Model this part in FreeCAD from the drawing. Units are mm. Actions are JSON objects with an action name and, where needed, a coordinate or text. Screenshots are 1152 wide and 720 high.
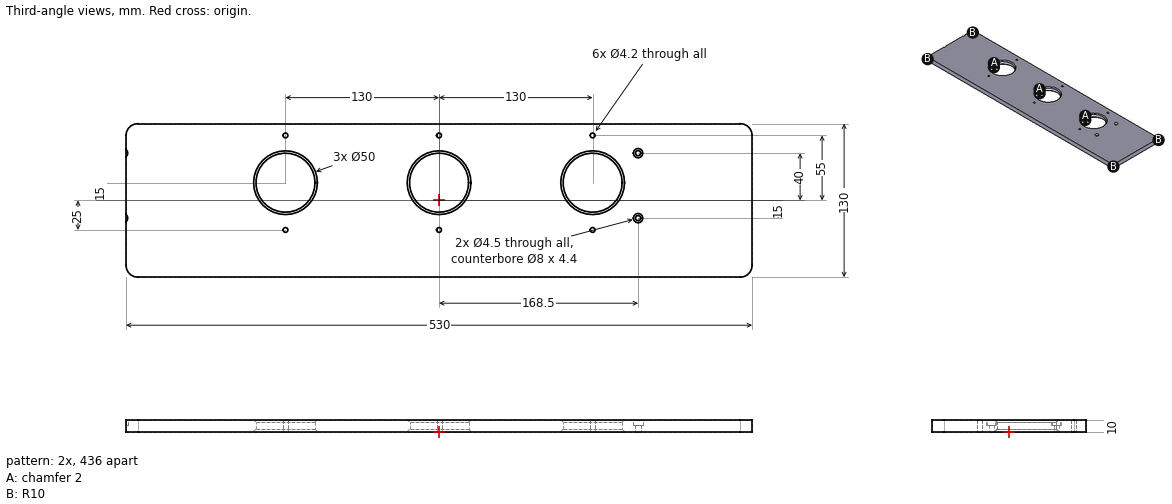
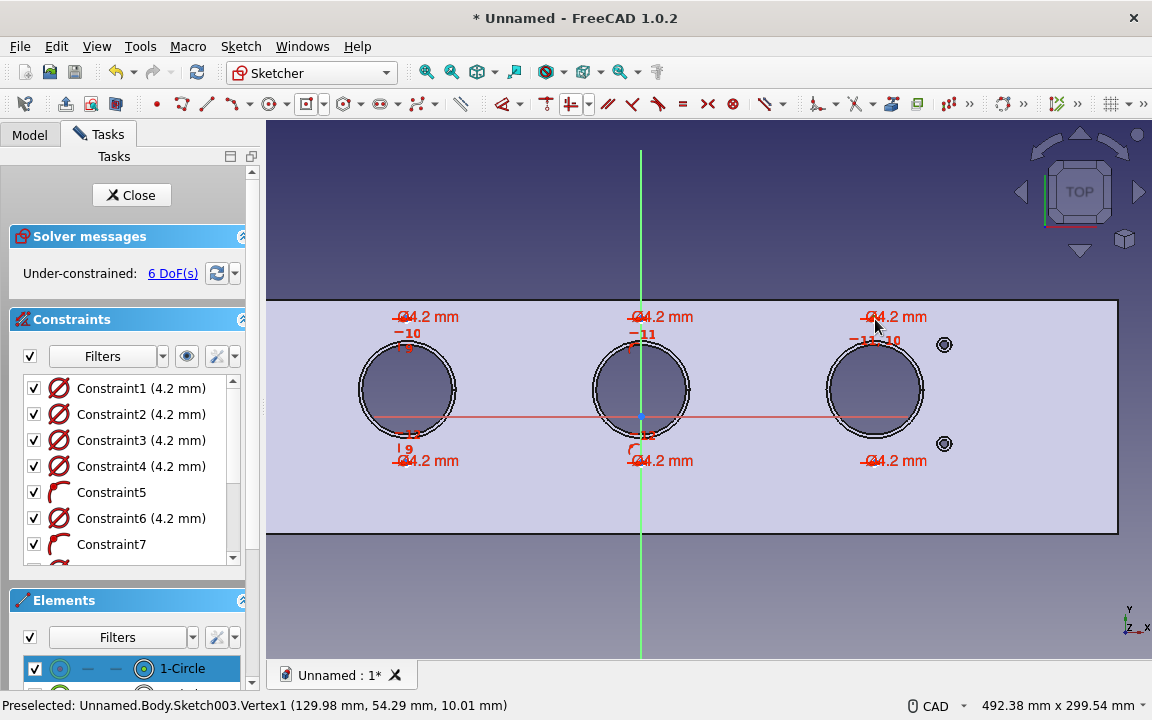
{"action": "left_click", "coordinate": [875, 463]}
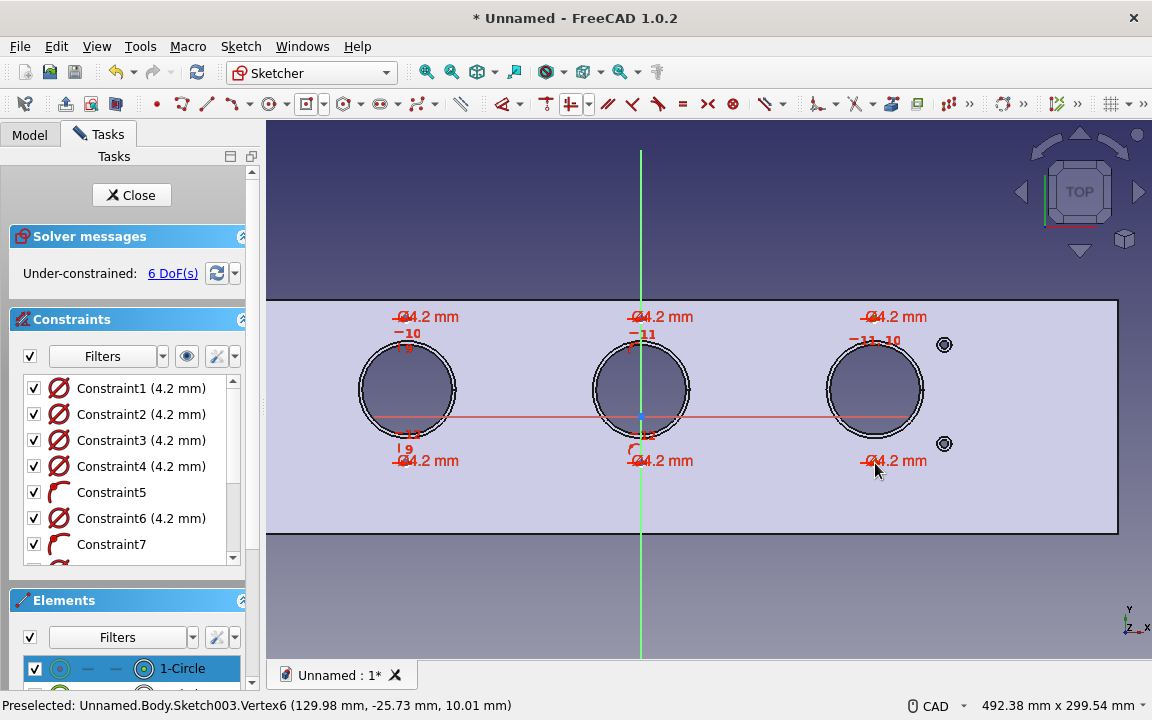
{"action": "left_click", "coordinate": [588, 104]}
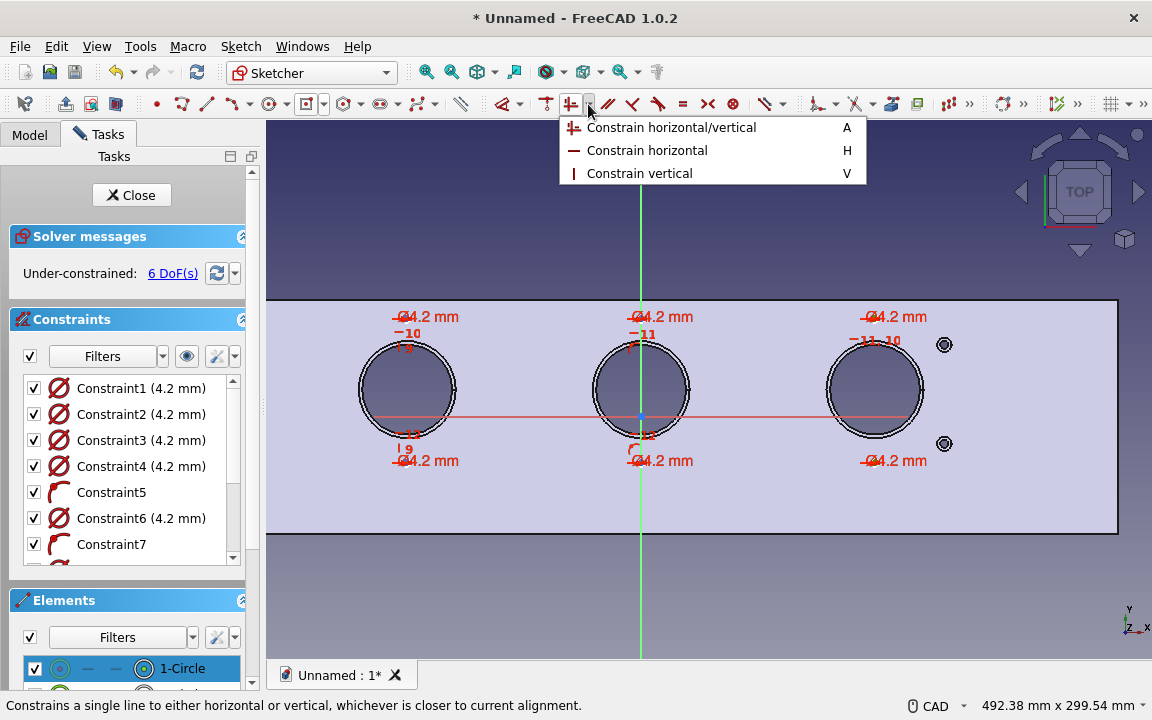
{"action": "left_click", "coordinate": [713, 174]}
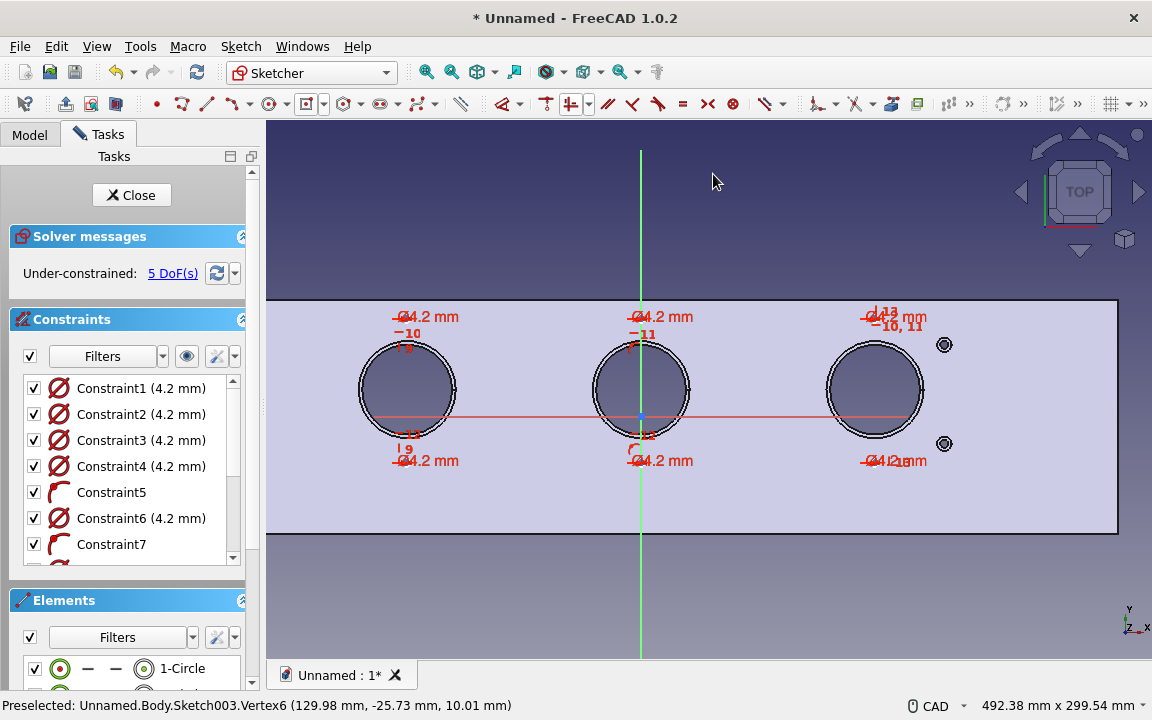
{"action": "left_click", "coordinate": [641, 463]}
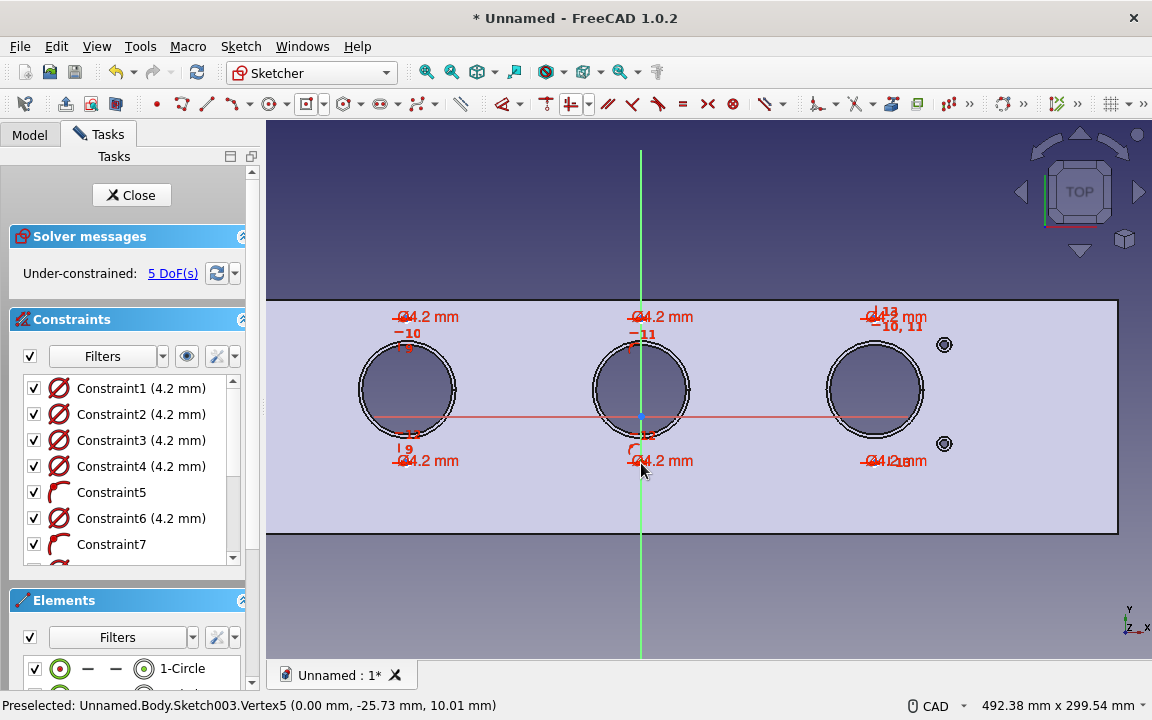
{"action": "left_click", "coordinate": [875, 463]}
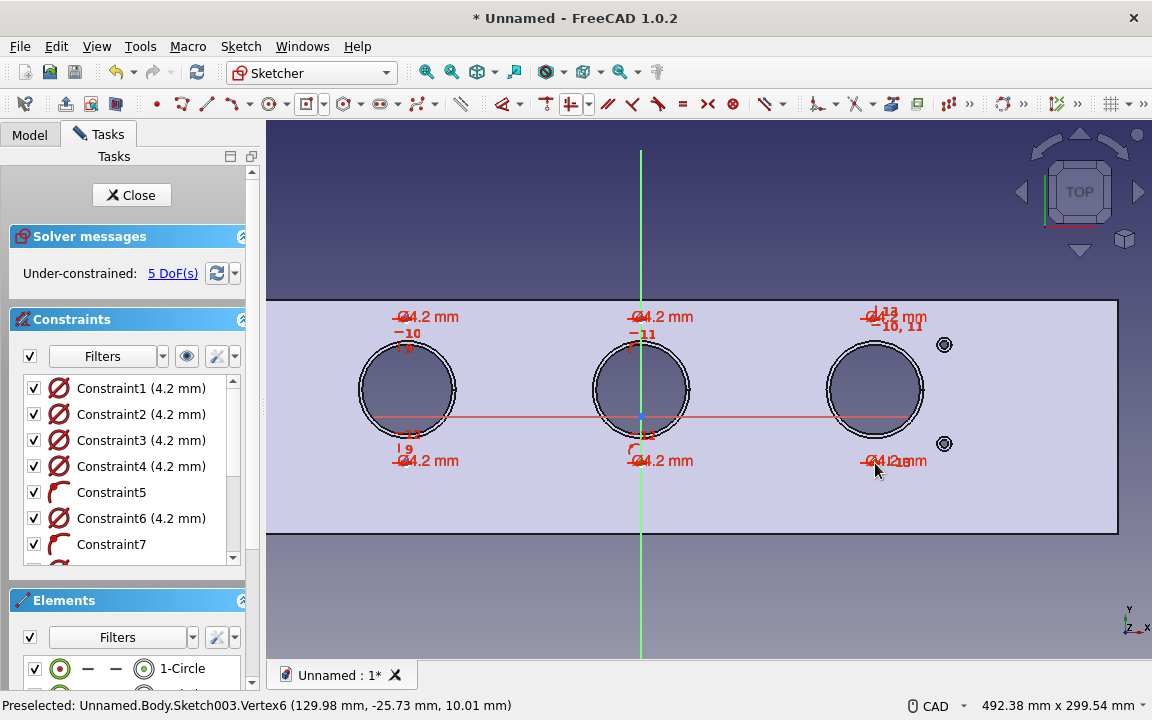
{"action": "left_click", "coordinate": [588, 104]}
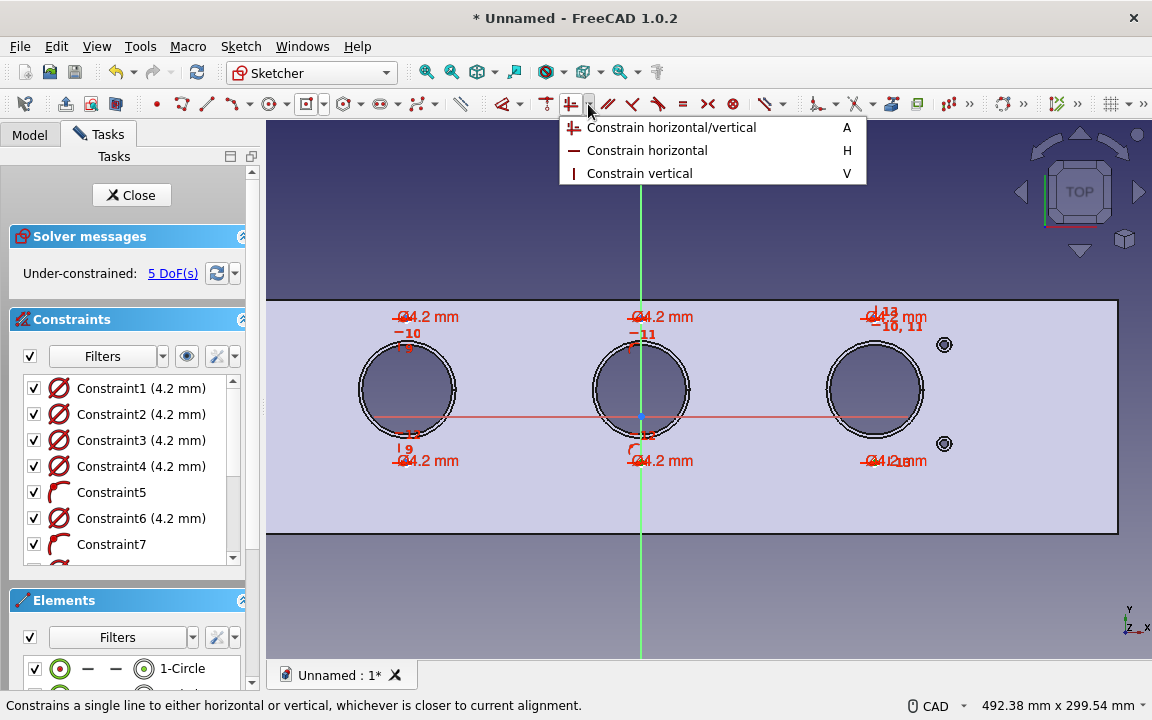
{"action": "left_click", "coordinate": [713, 150]}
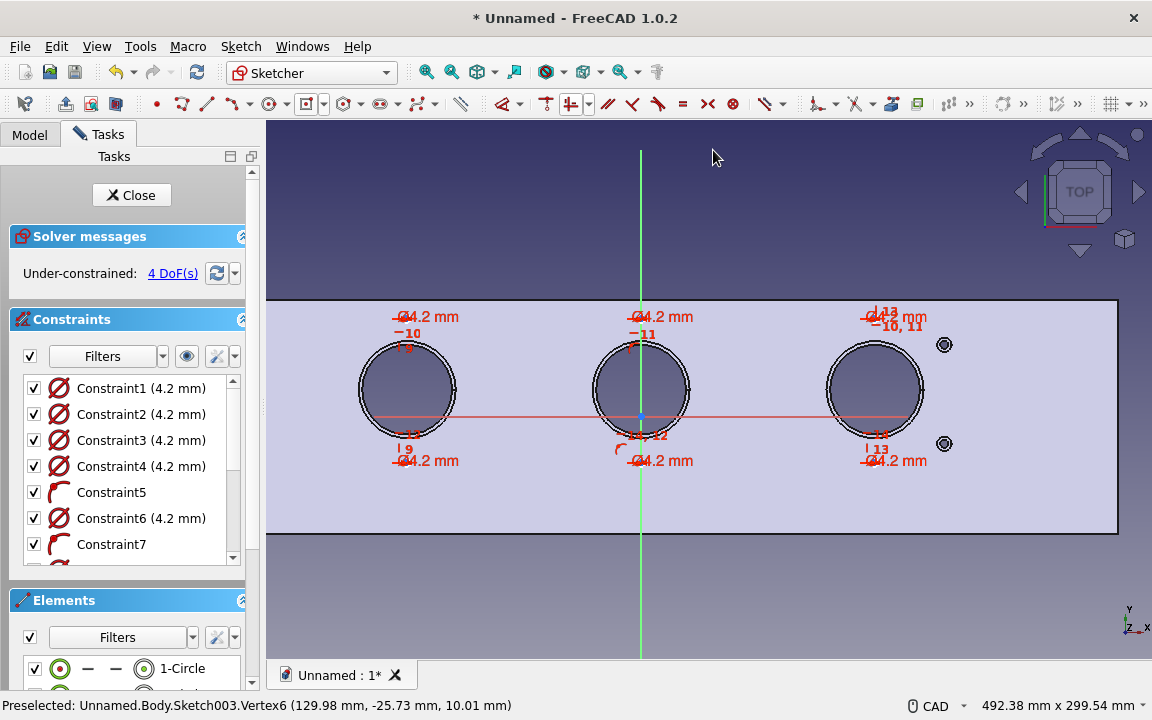
{"action": "left_click", "coordinate": [502, 104]}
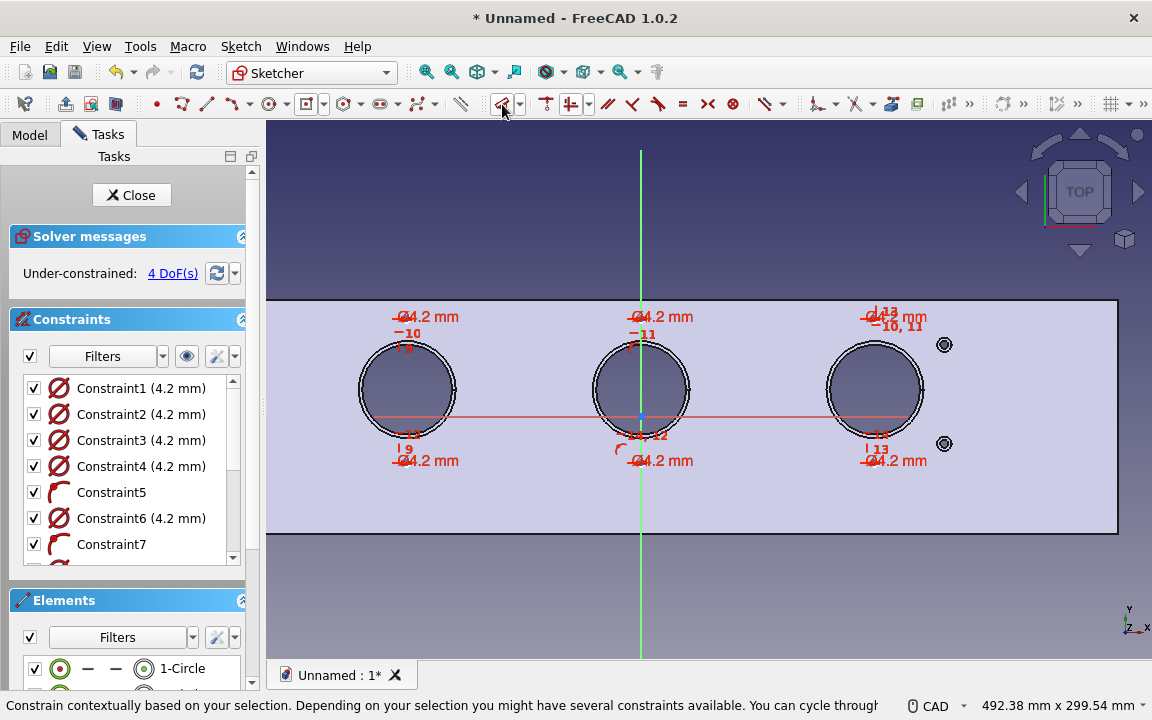
{"action": "left_click", "coordinate": [875, 319]}
{"action": "left_click", "coordinate": [909, 368]}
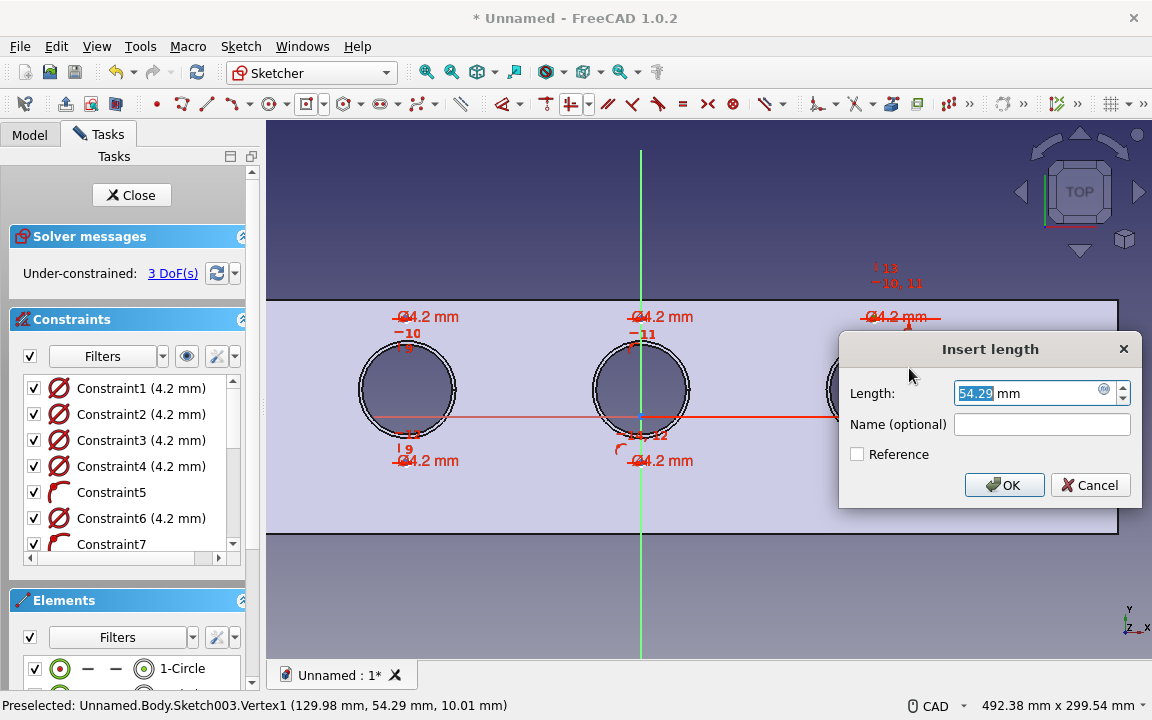
{"action": "type", "text": "55"}
{"action": "key", "text": "Return"}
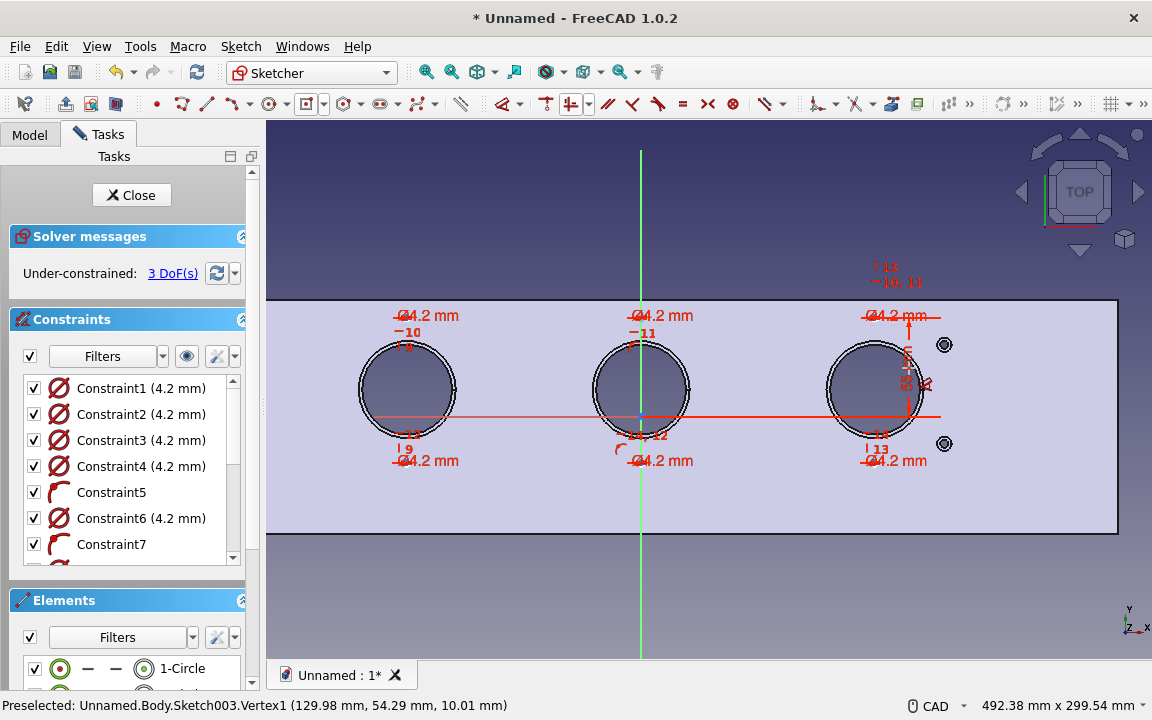
{"action": "left_click", "coordinate": [407, 463]}
{"action": "left_click", "coordinate": [373, 440]}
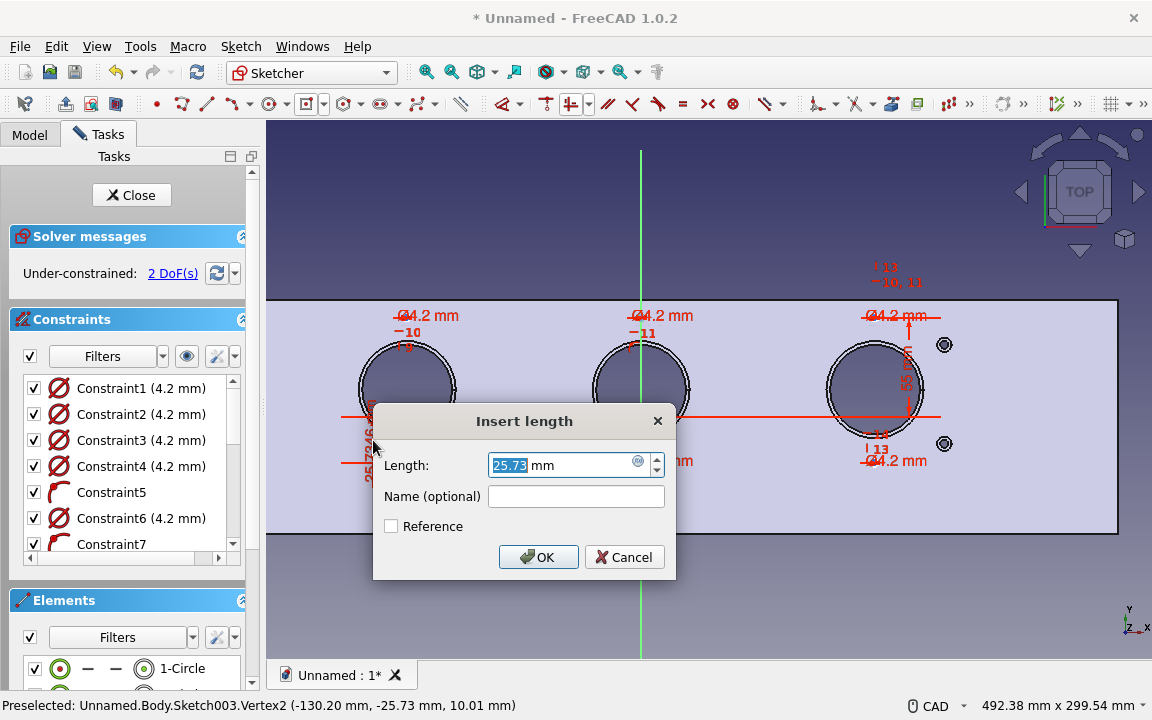
{"action": "type", "text": "25"}
{"action": "key", "text": "Return"}